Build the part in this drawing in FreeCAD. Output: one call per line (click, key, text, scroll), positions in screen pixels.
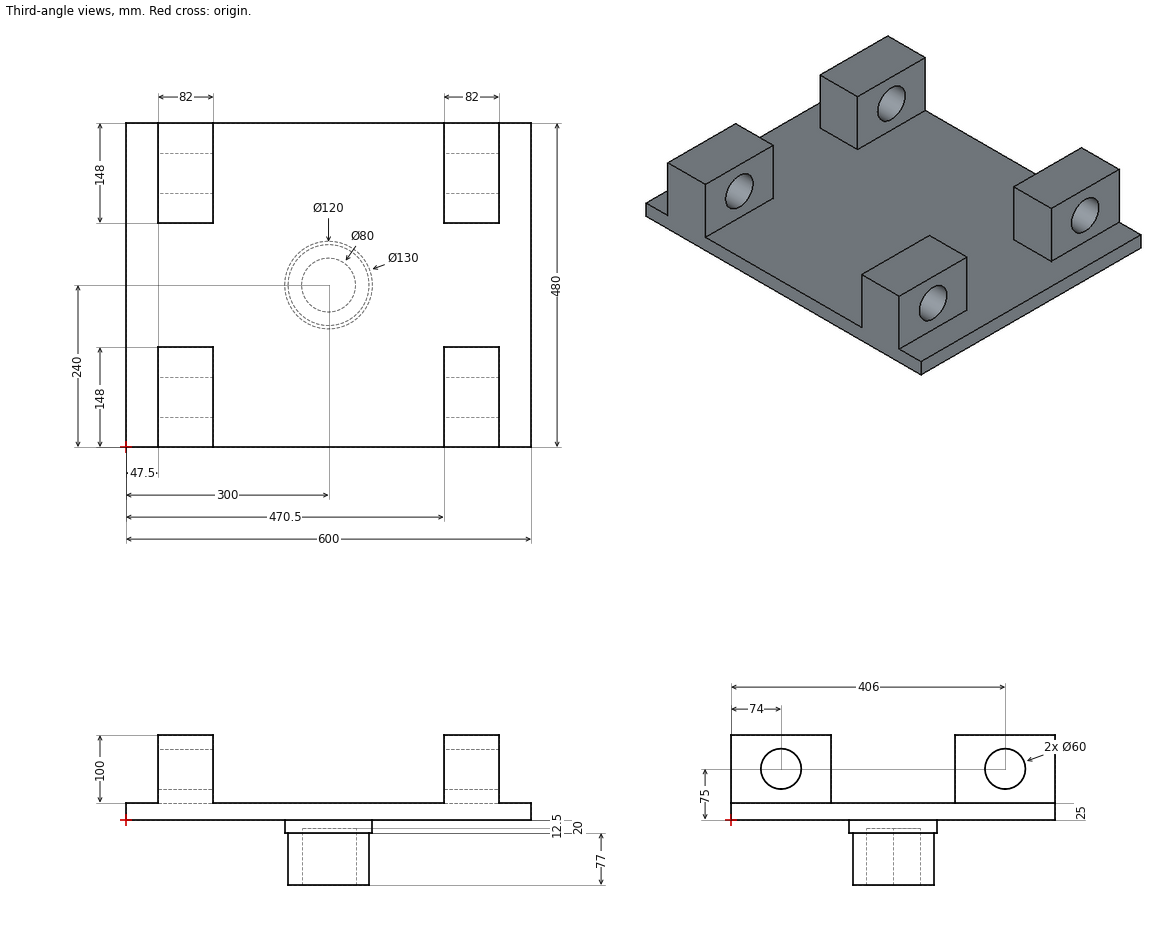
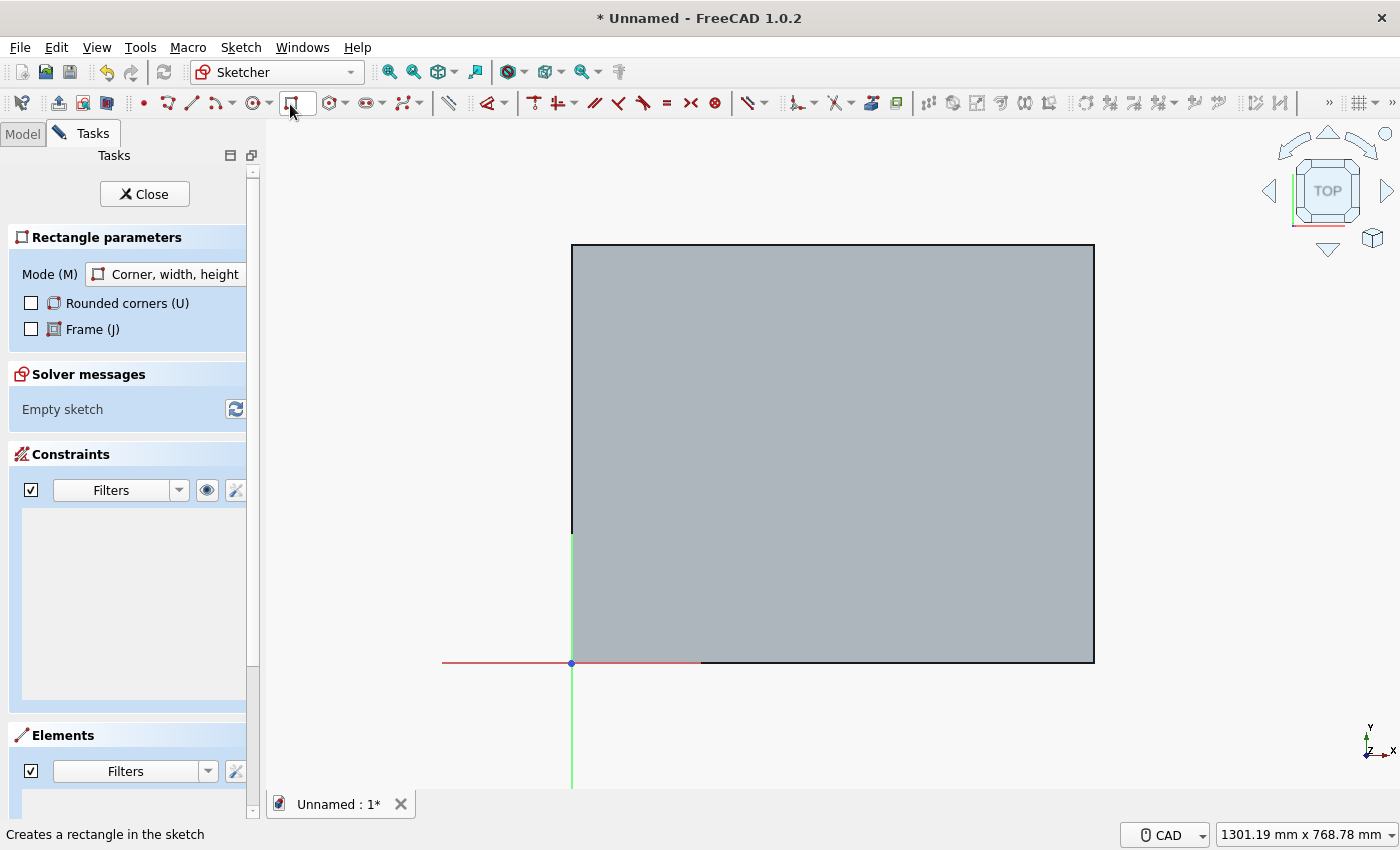
click(613, 245)
move(684, 374)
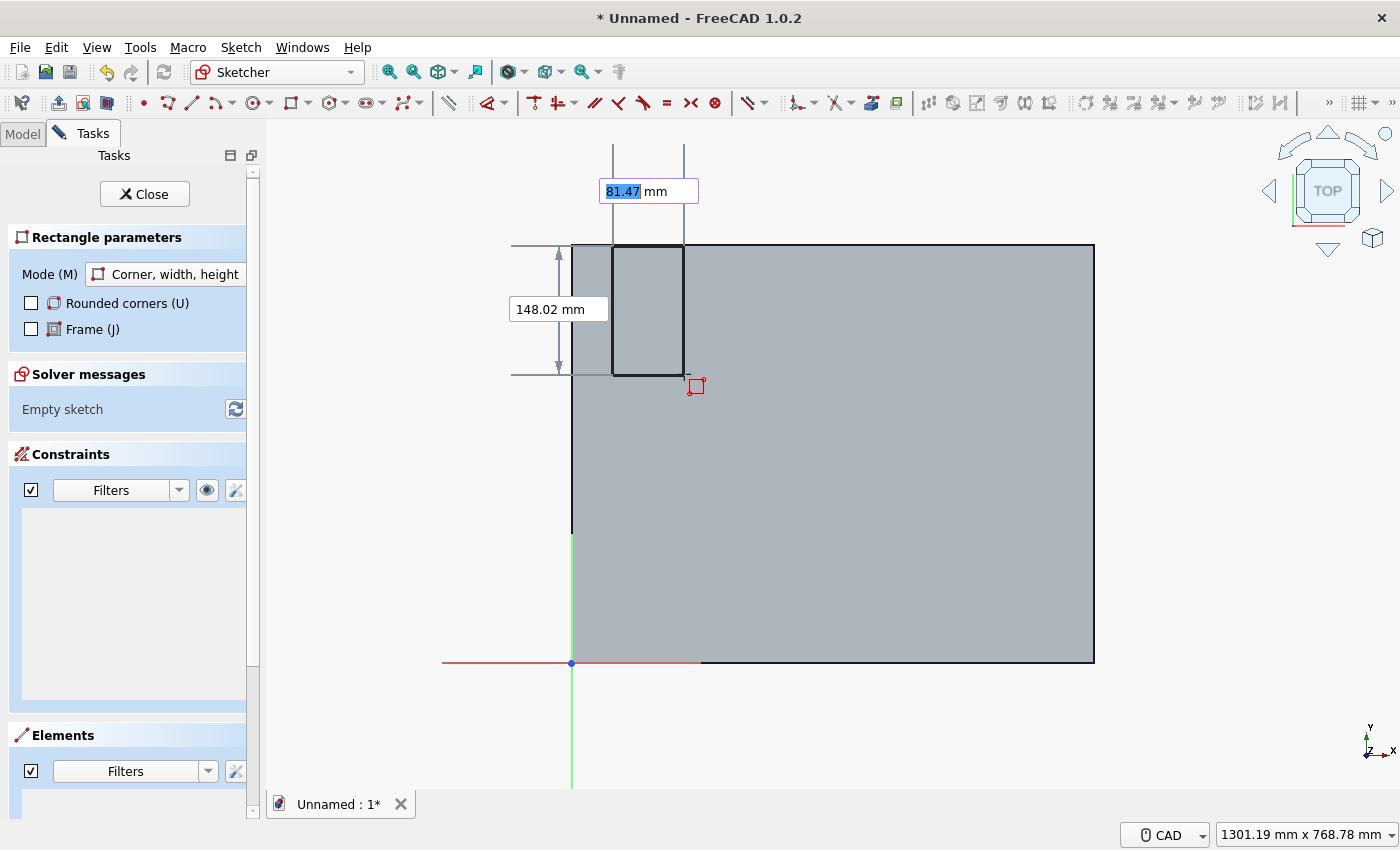
text(82)
key(Tab)
text(148)
key(Return)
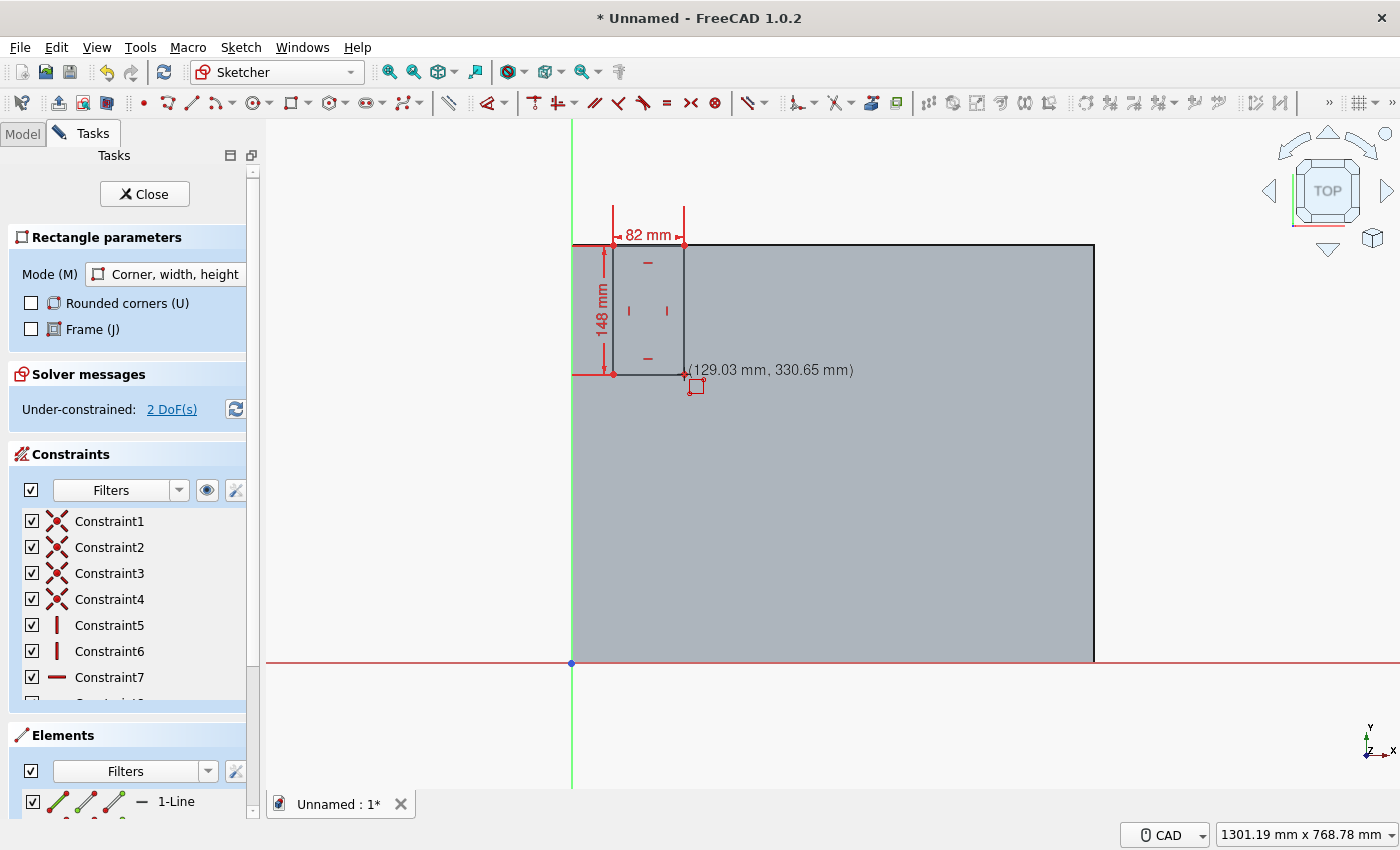
click(613, 534)
click(684, 663)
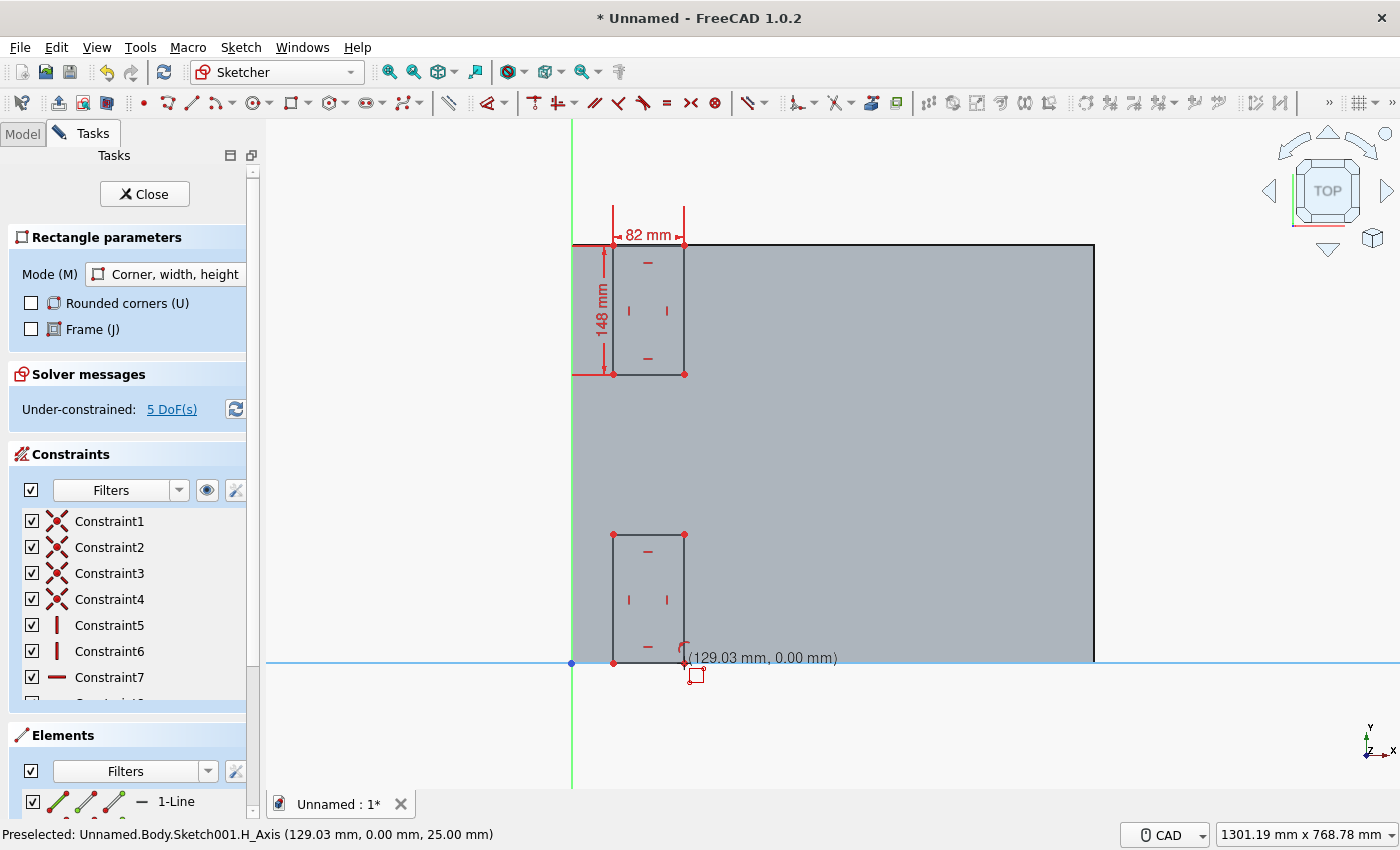
click(982, 534)
click(1053, 663)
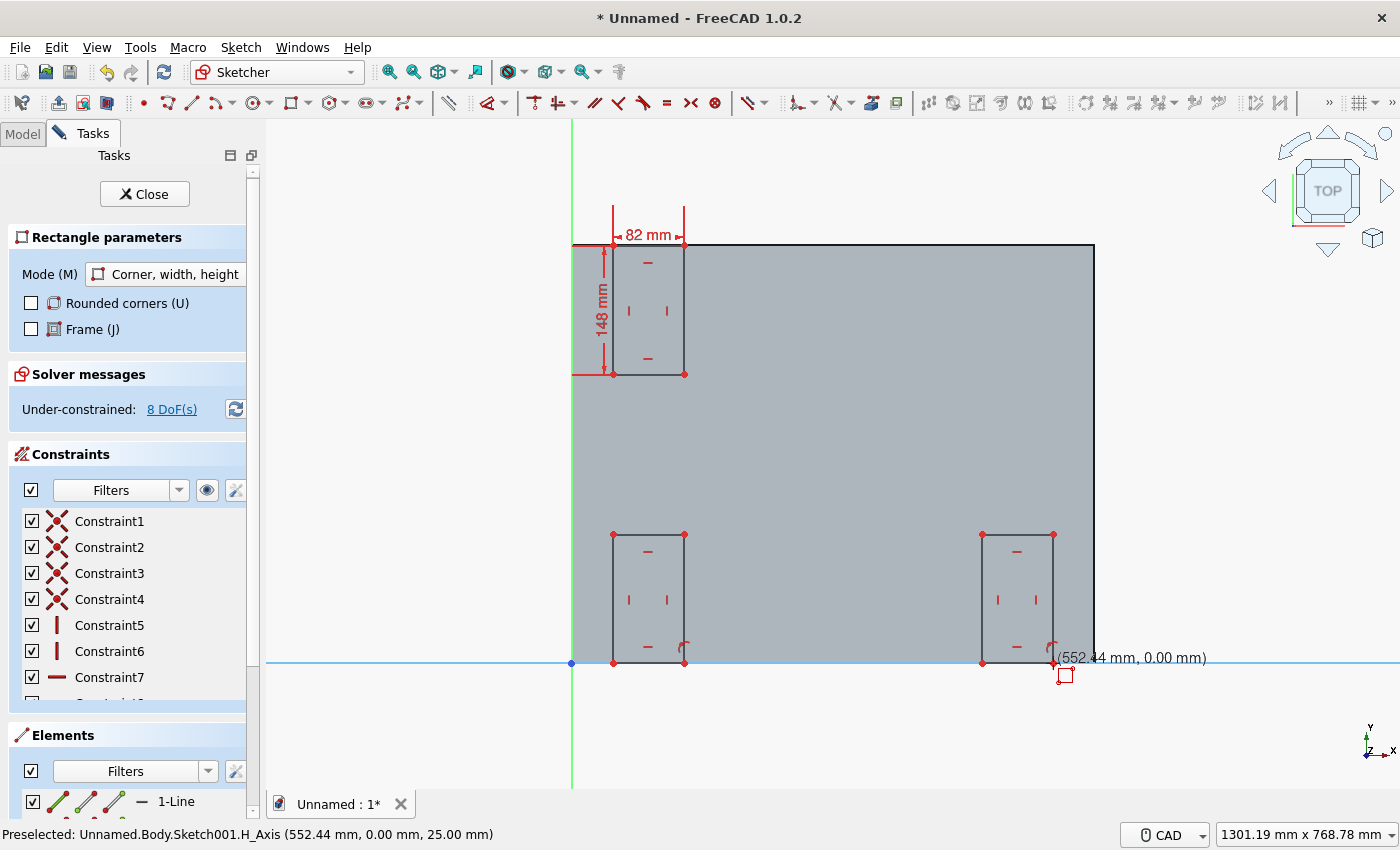
click(982, 245)
move(1053, 374)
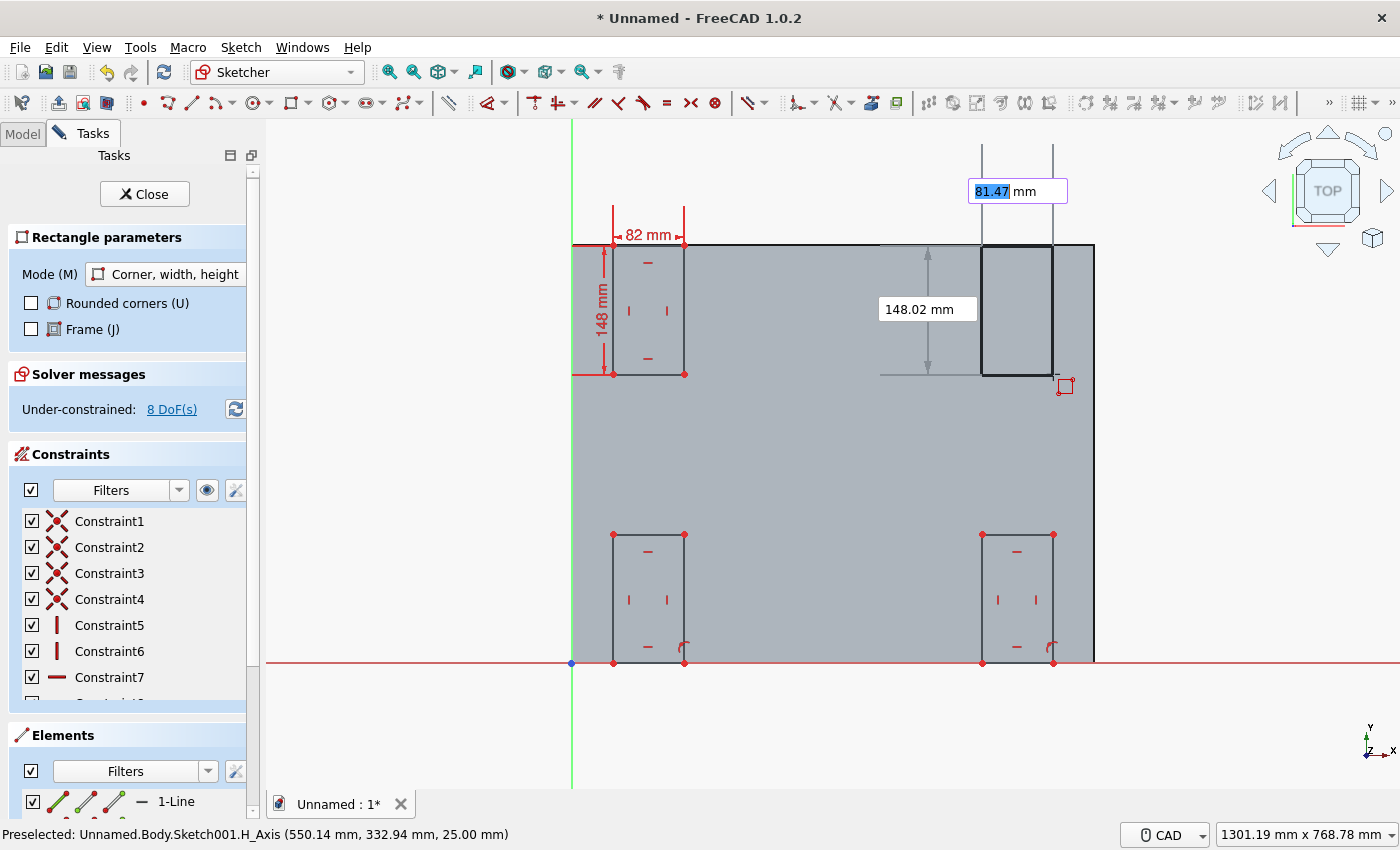
text(82)
key(Tab)
text(148)
key(Return)
key(Escape)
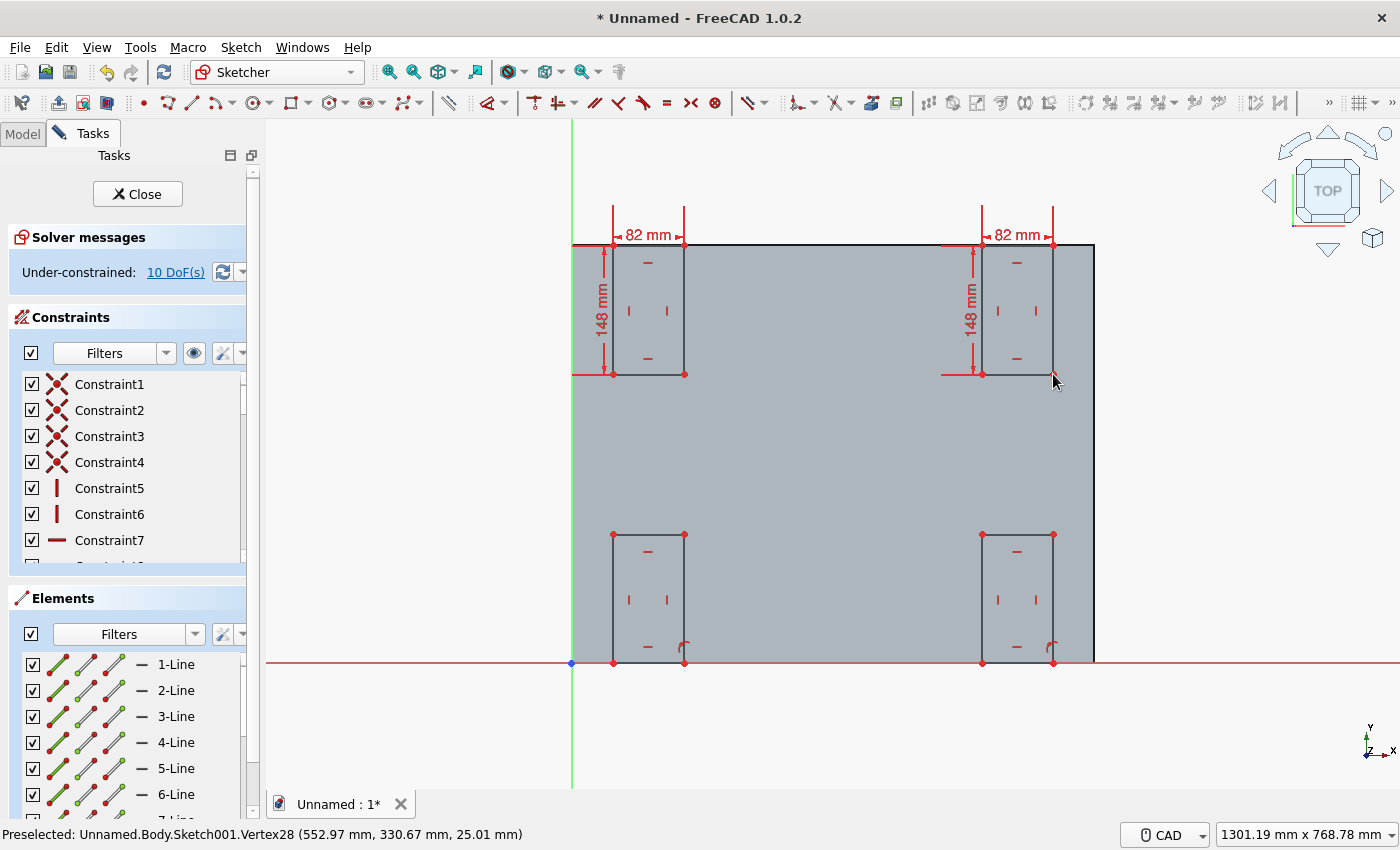
key(d)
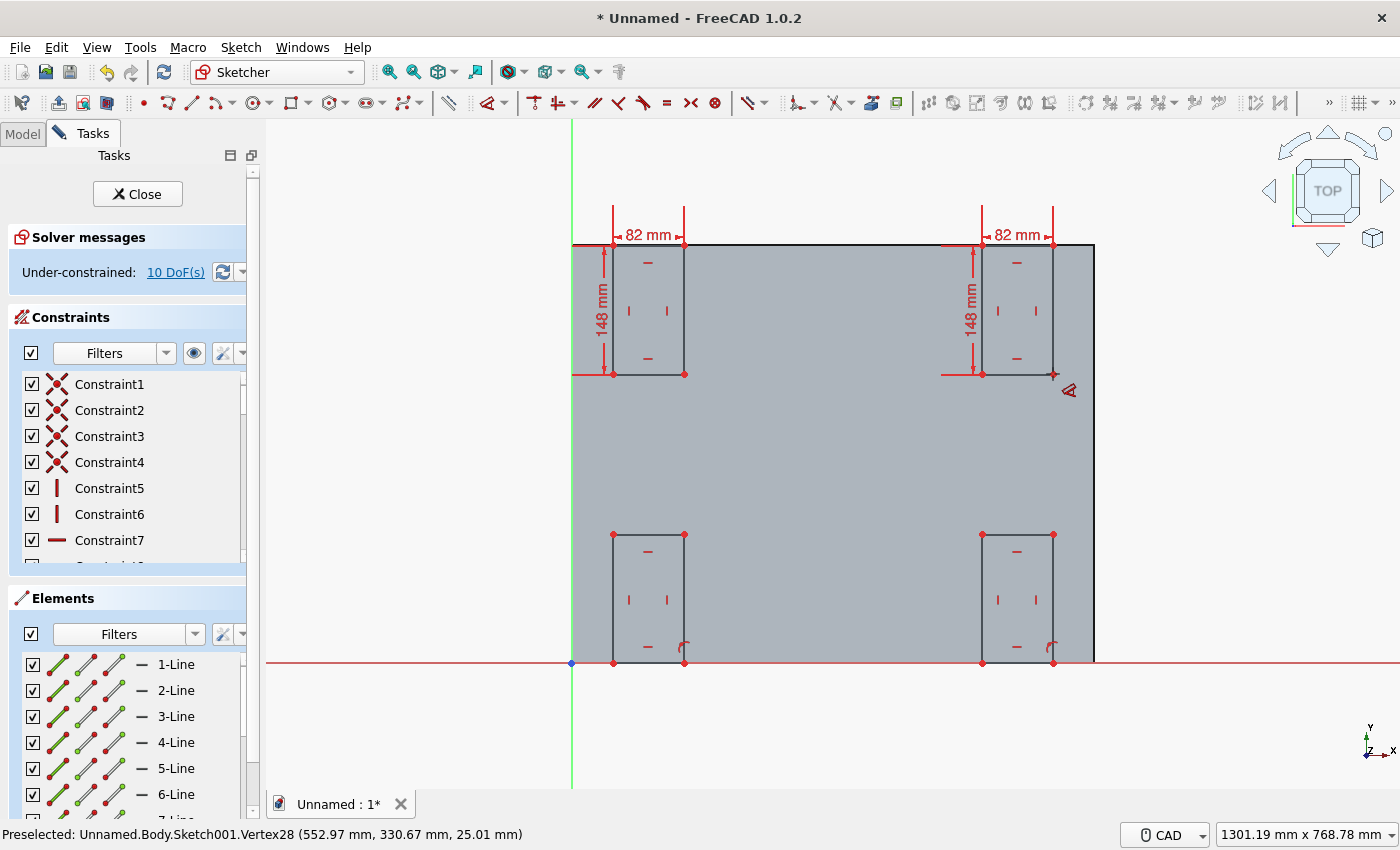
click(634, 663)
click(649, 697)